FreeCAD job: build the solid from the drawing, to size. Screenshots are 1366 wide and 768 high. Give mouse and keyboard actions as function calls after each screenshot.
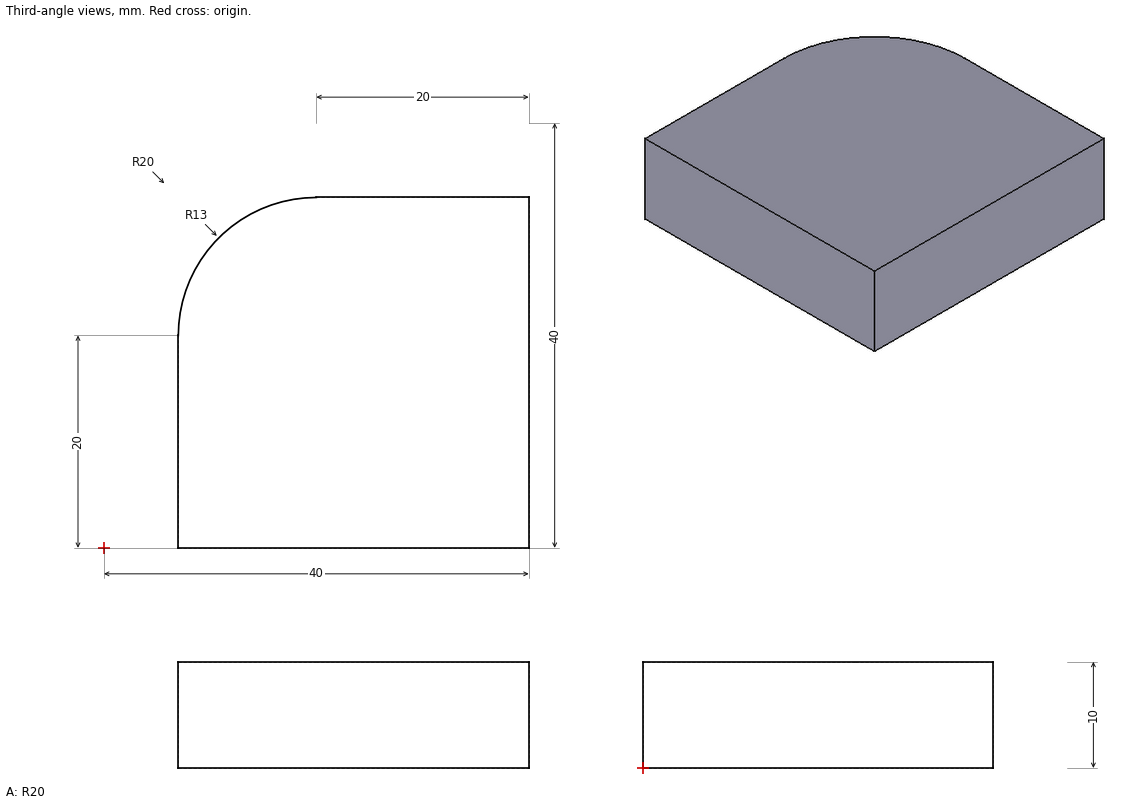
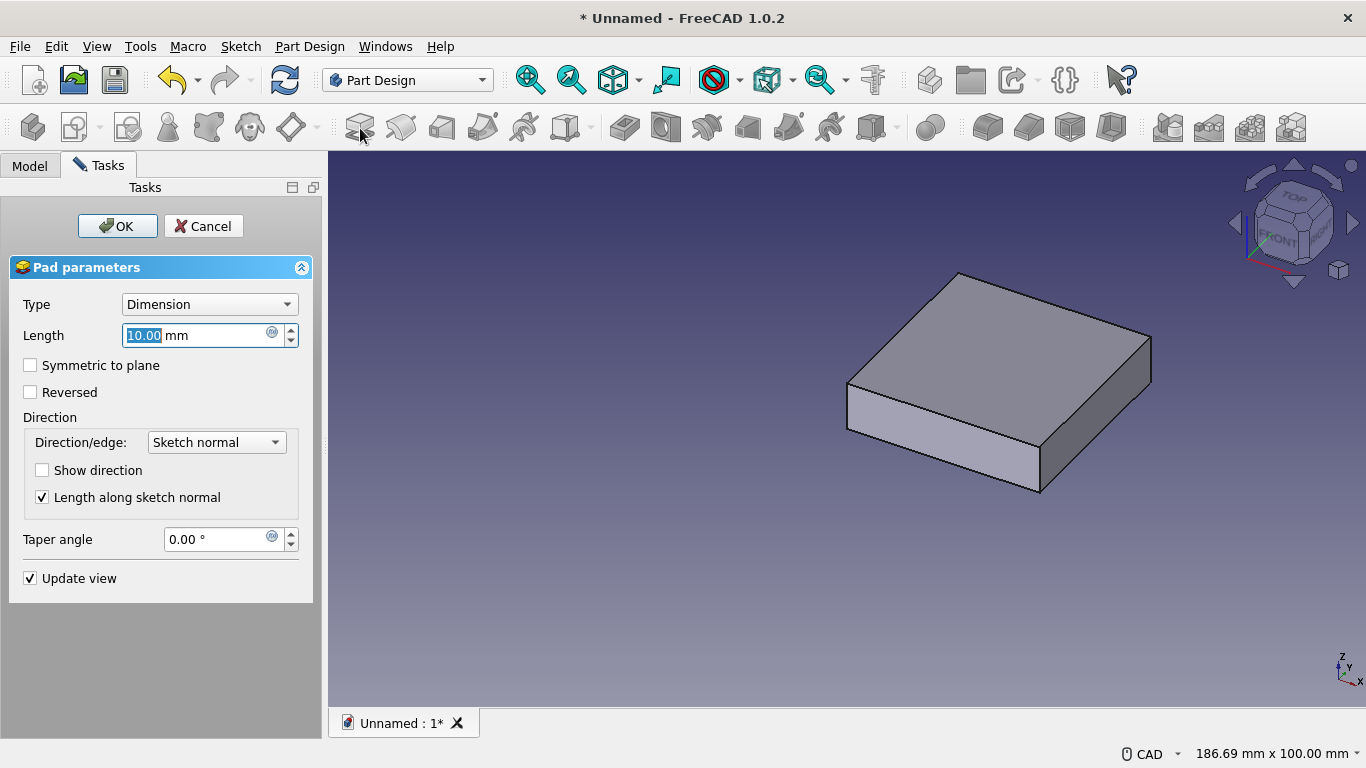
text(10)
key(Tab)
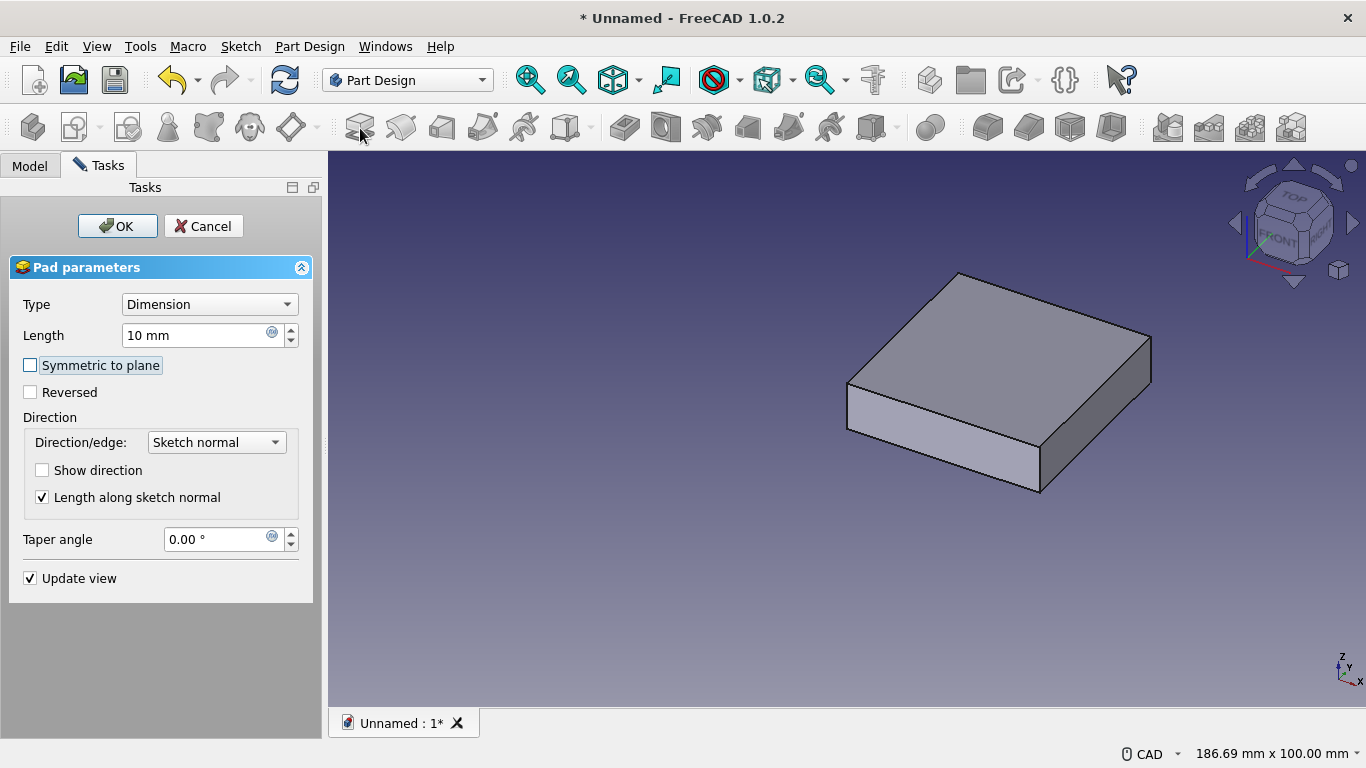
click(118, 226)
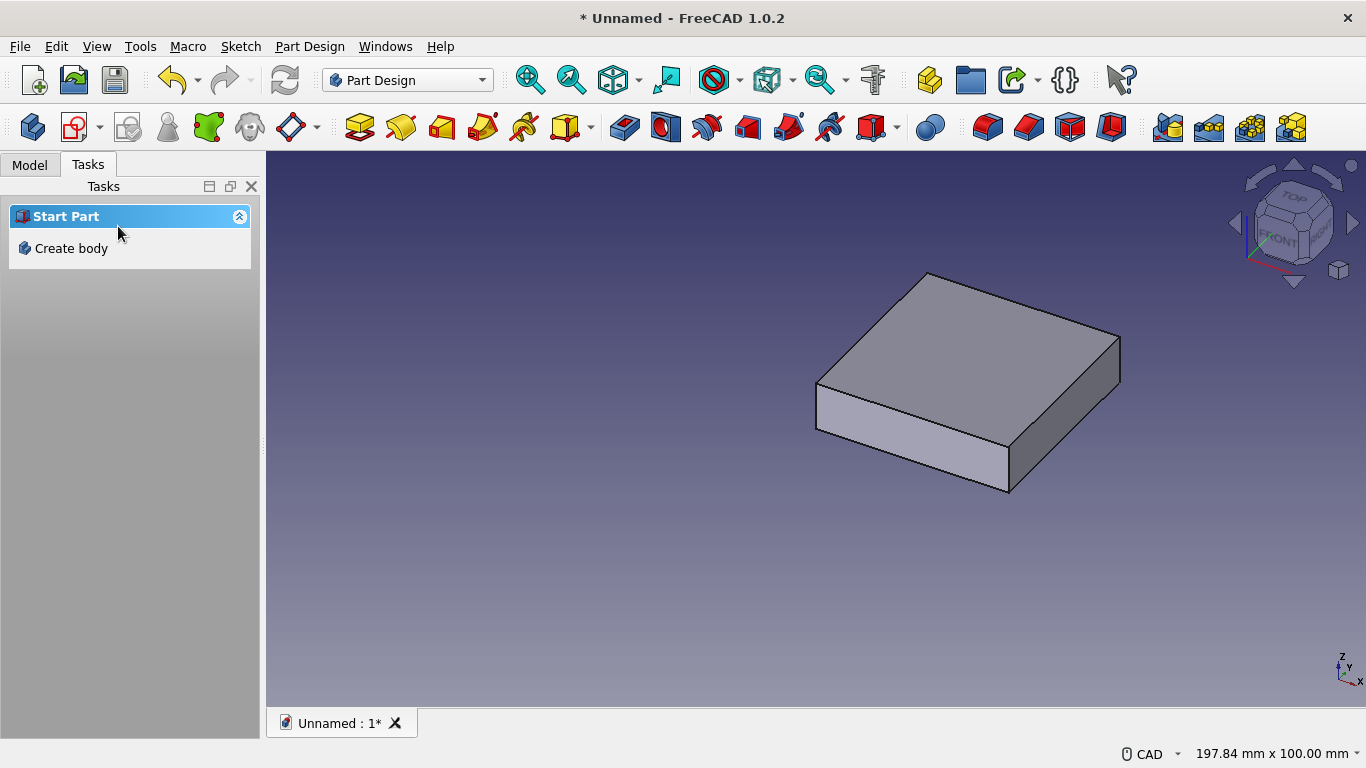
click(531, 80)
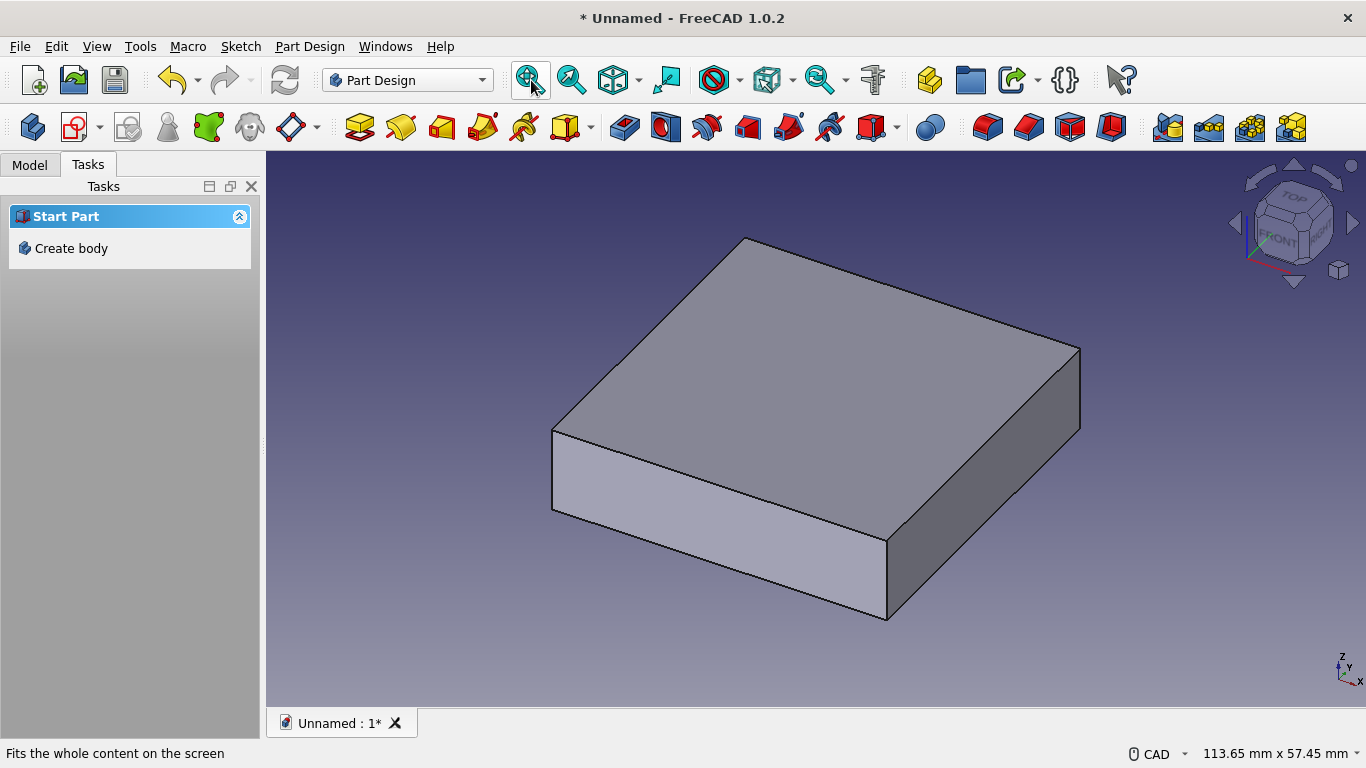
key(0)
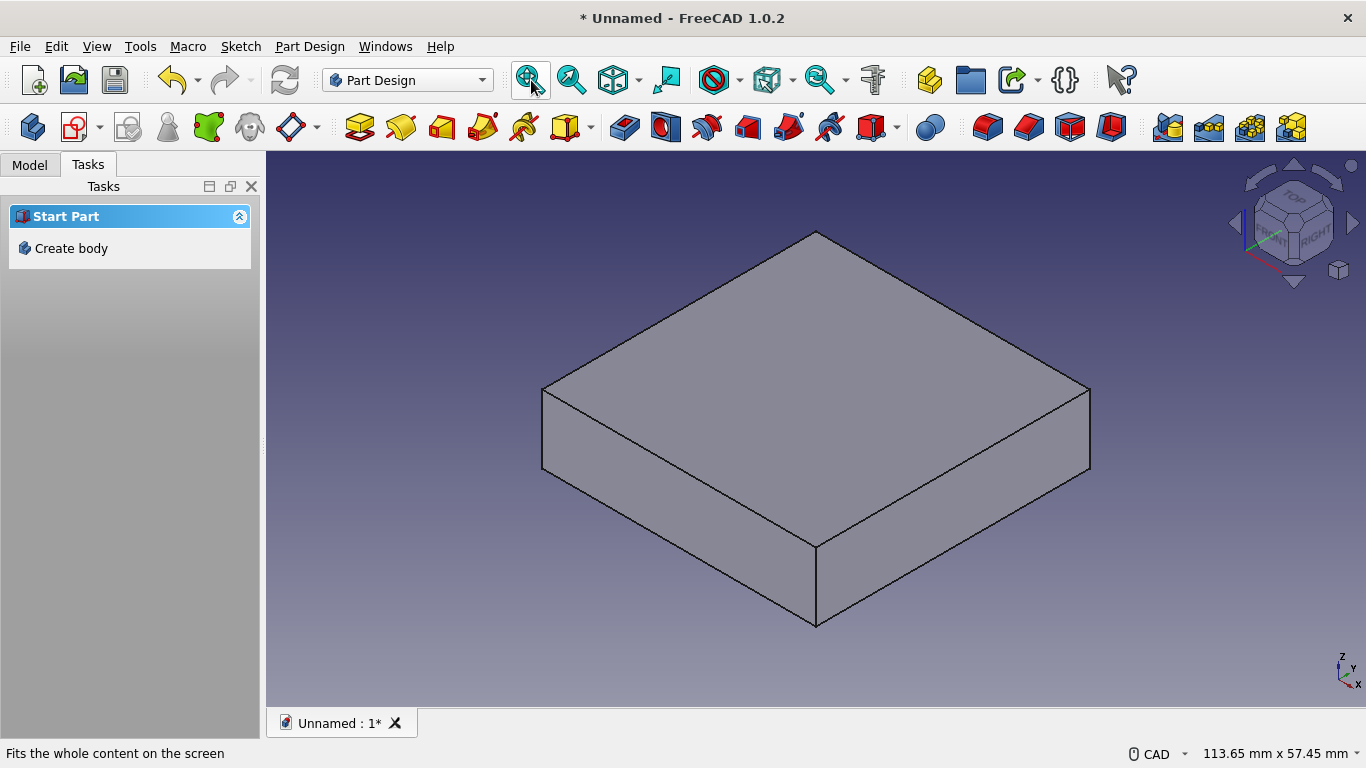
key(2)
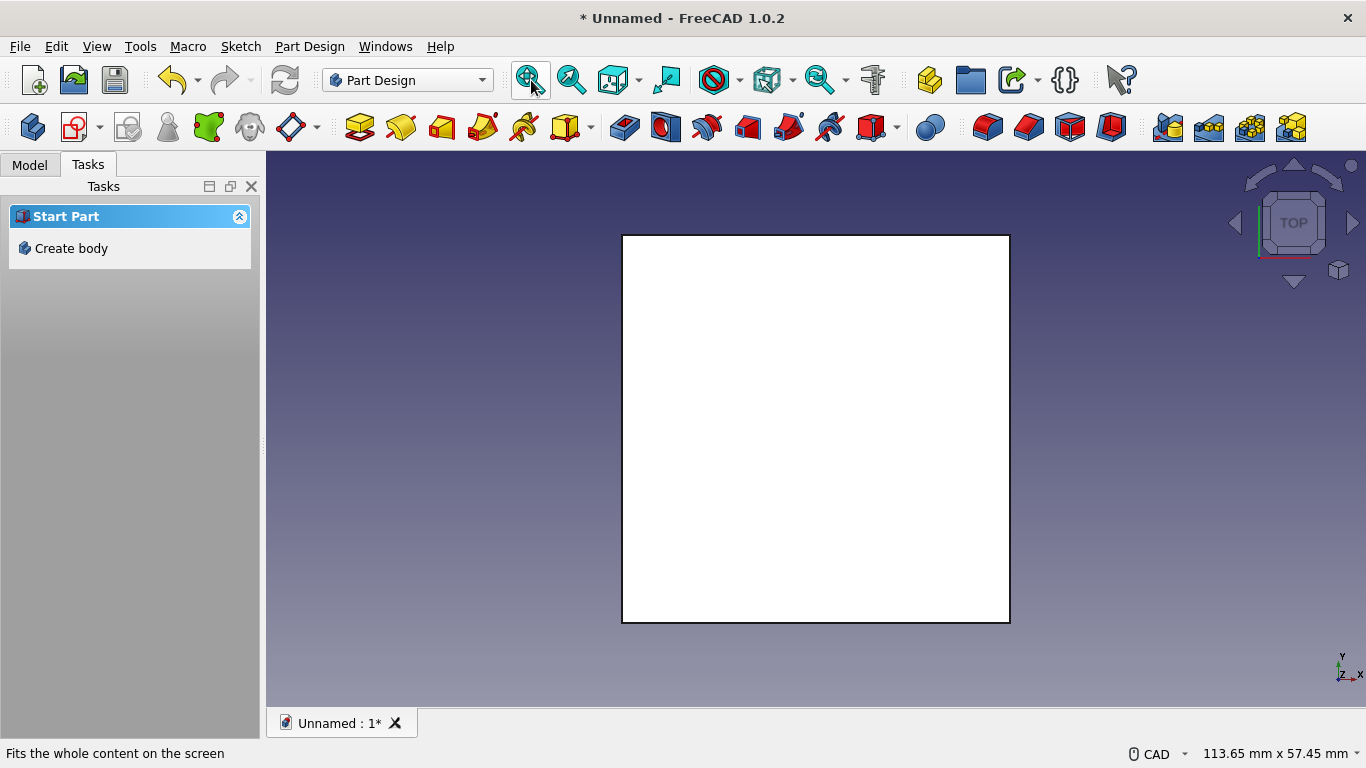
key(1)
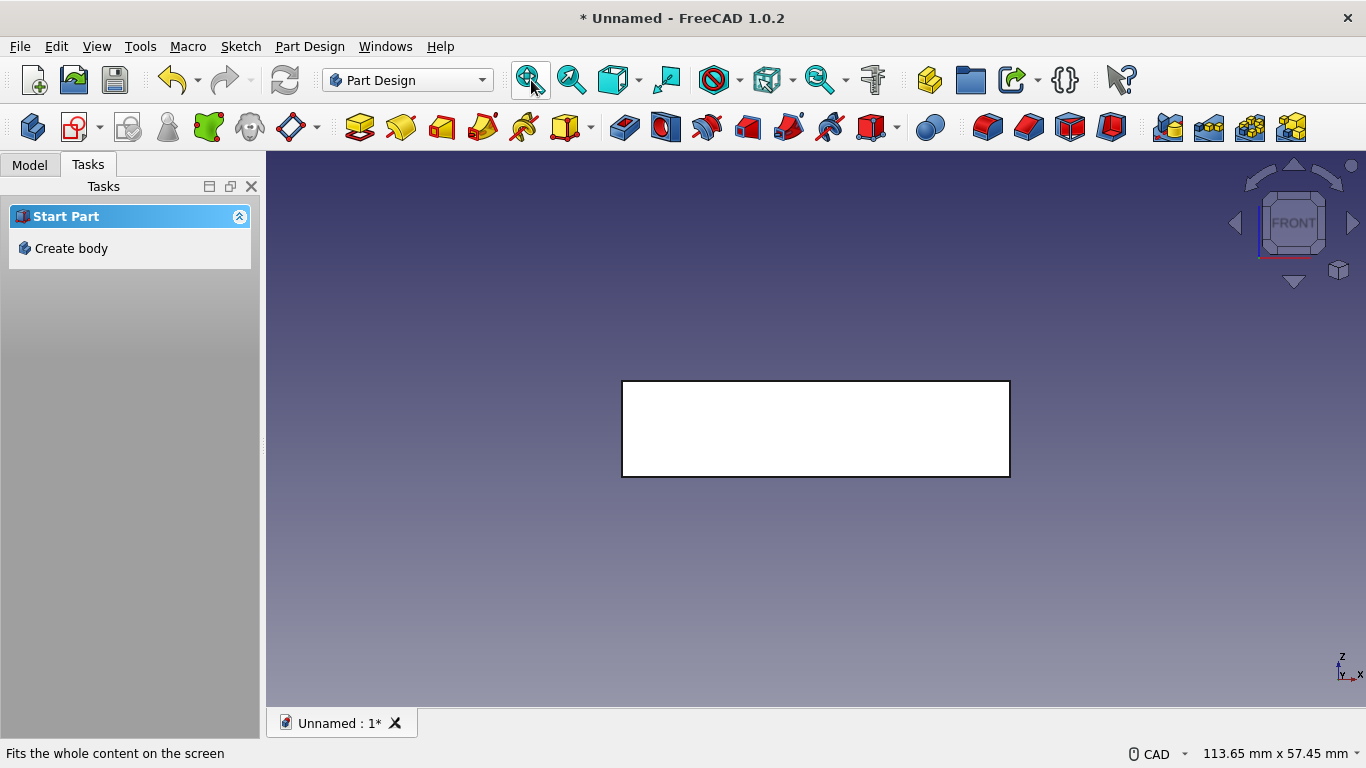
click(531, 80)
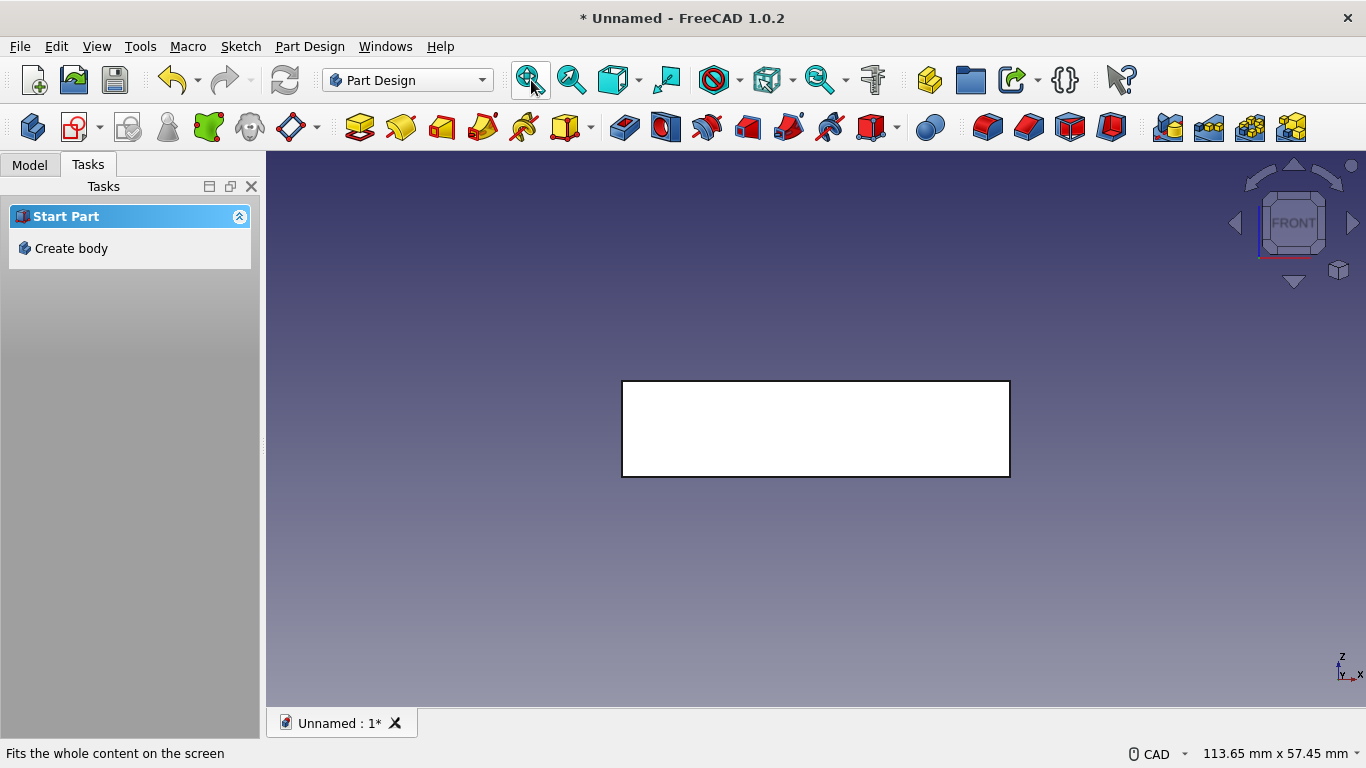
key(3)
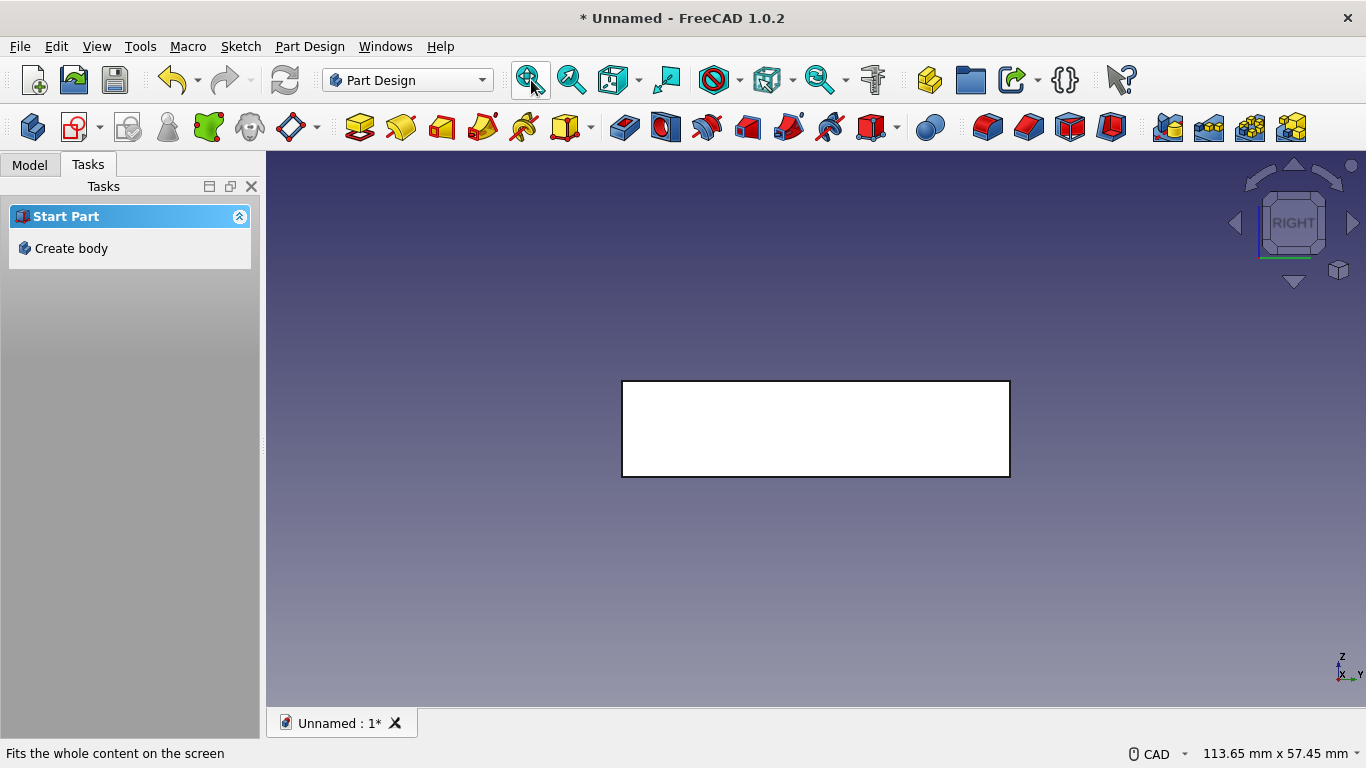
click(531, 80)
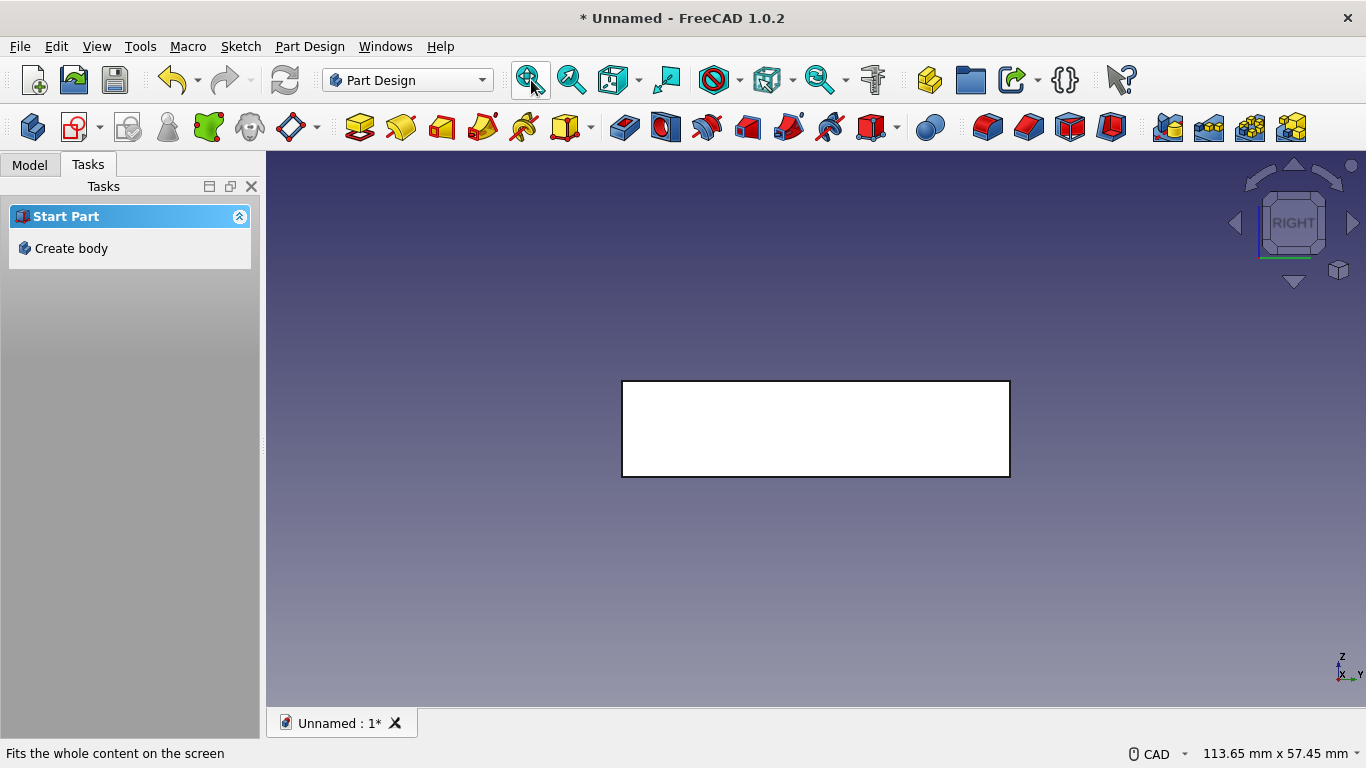
key(5)